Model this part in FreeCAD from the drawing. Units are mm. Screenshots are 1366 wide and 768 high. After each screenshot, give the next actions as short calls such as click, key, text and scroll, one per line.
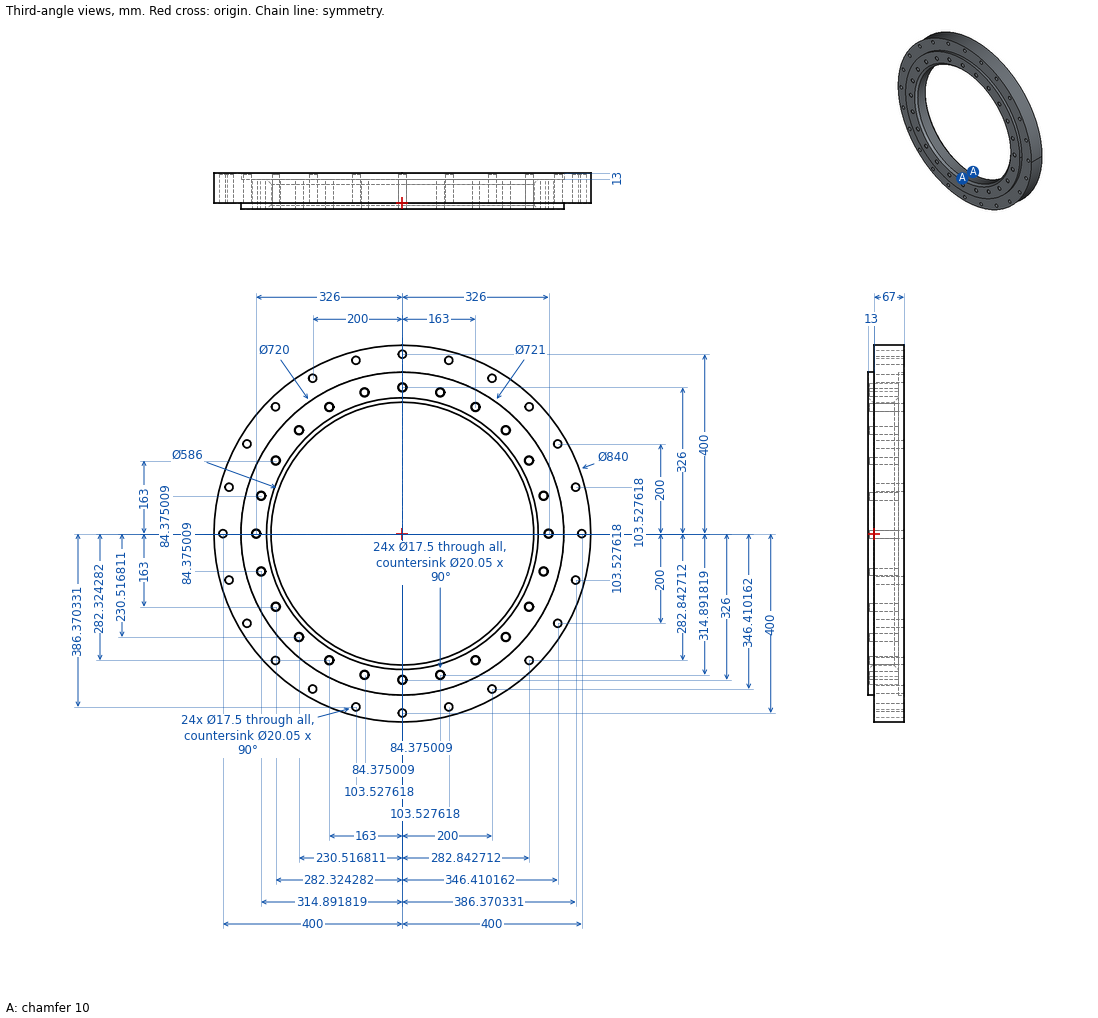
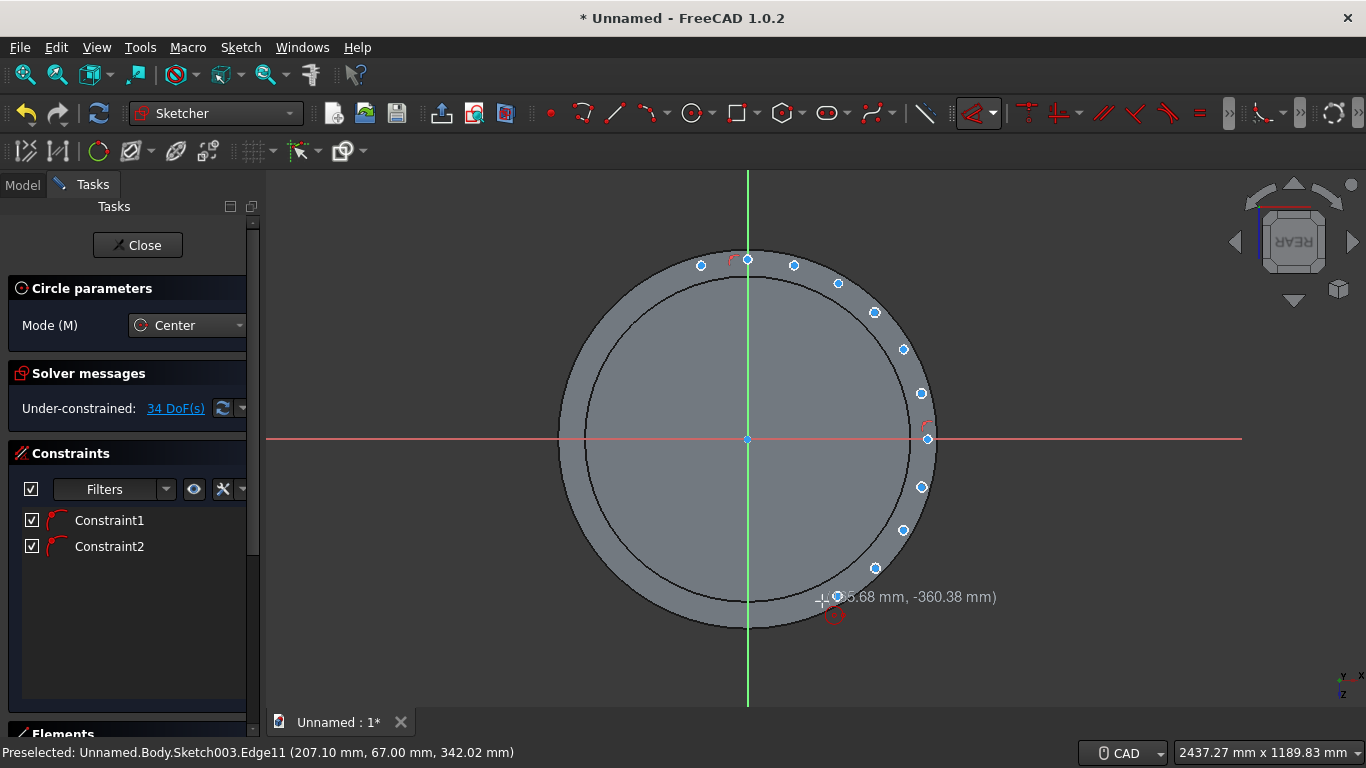
click(794, 614)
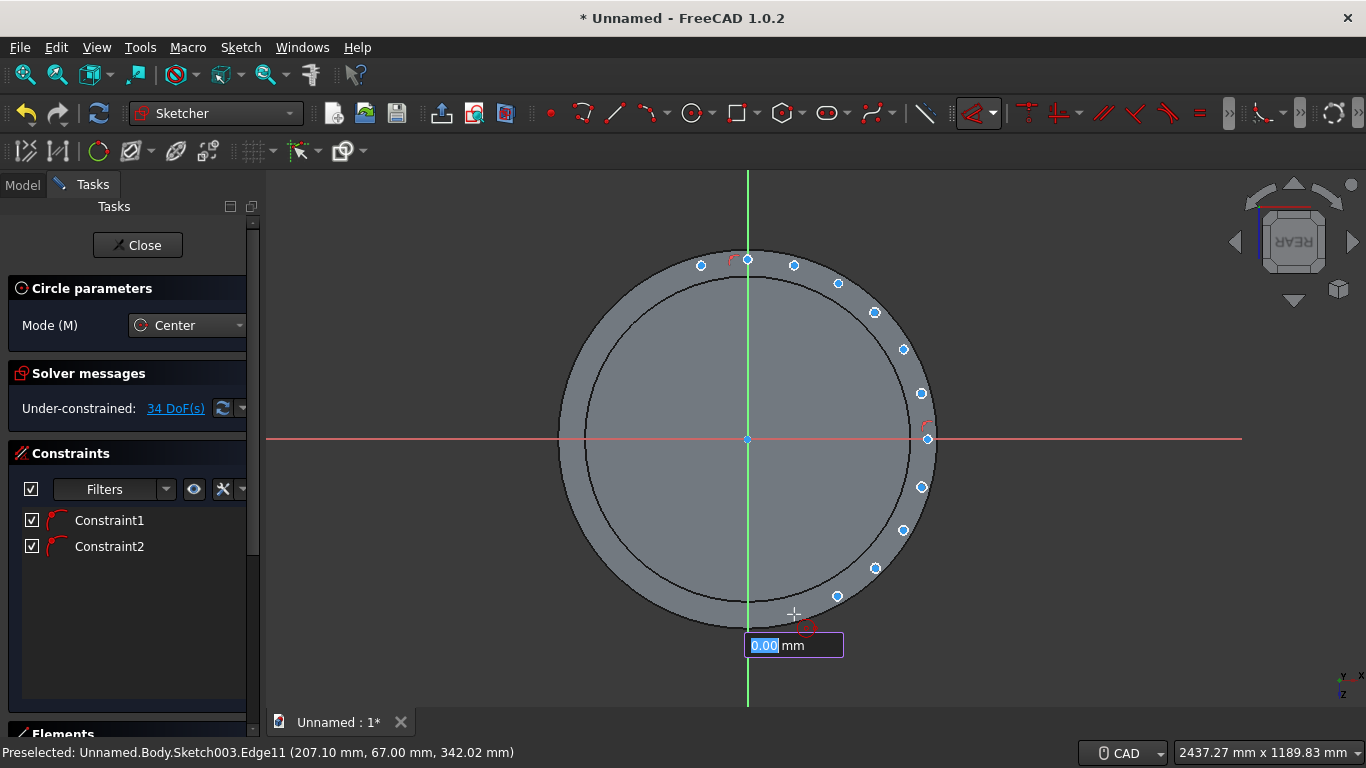
scroll(797, 611, up, 7)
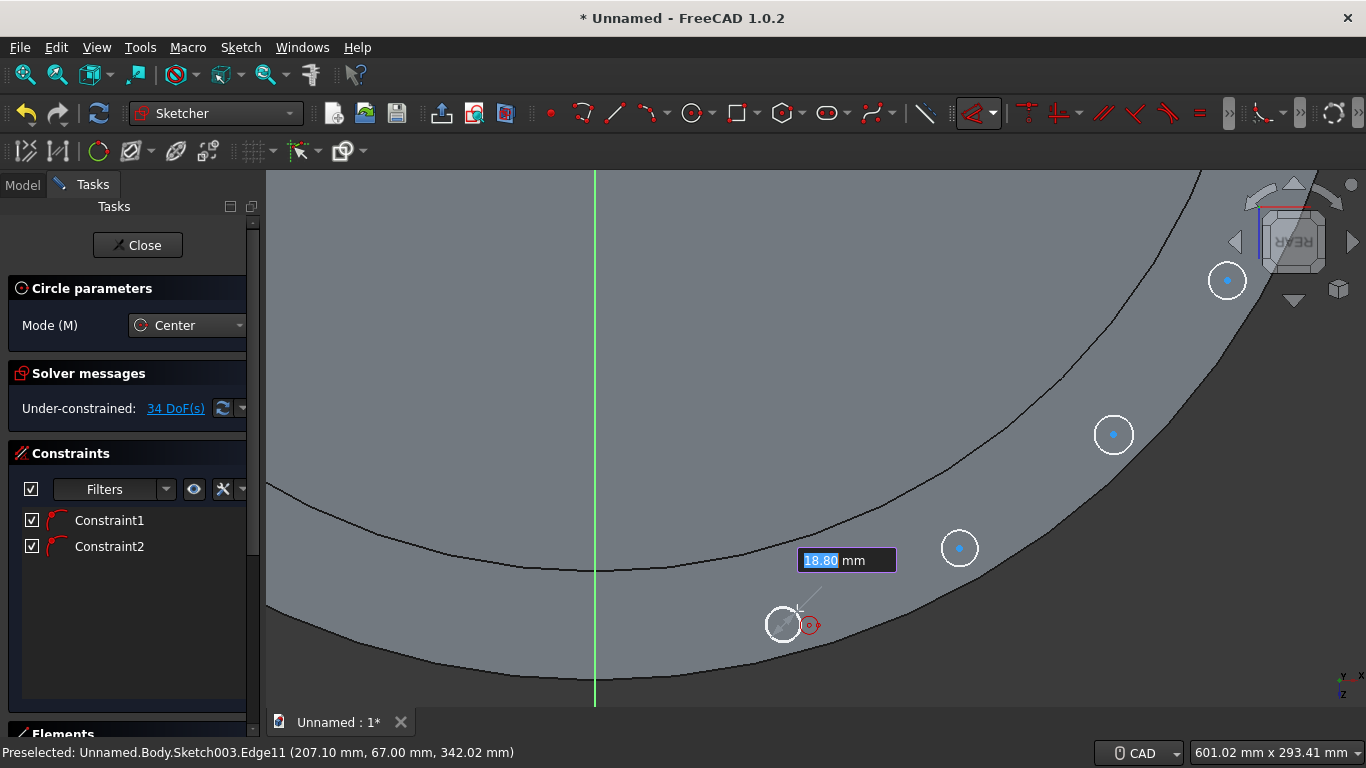
click(796, 608)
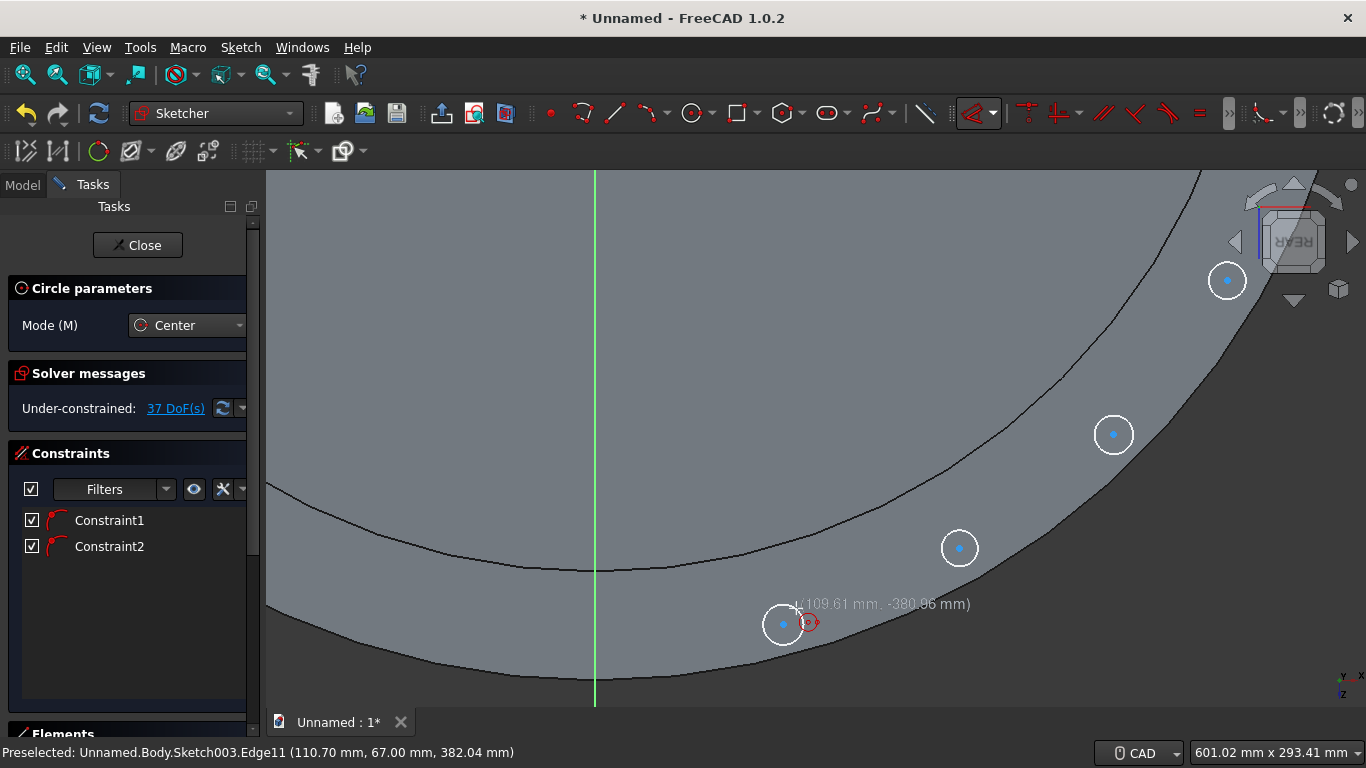
scroll(595, 644, up, 2)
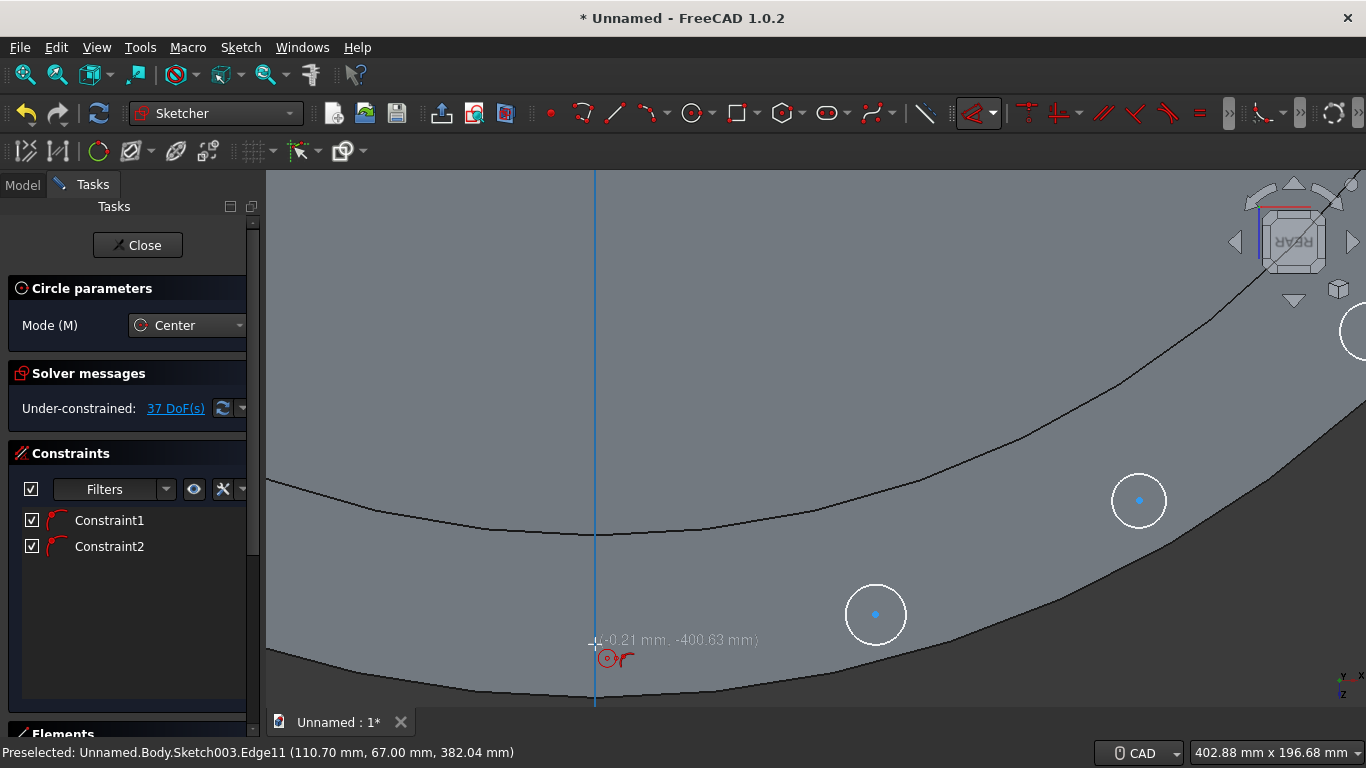
scroll(778, 614, down, 9)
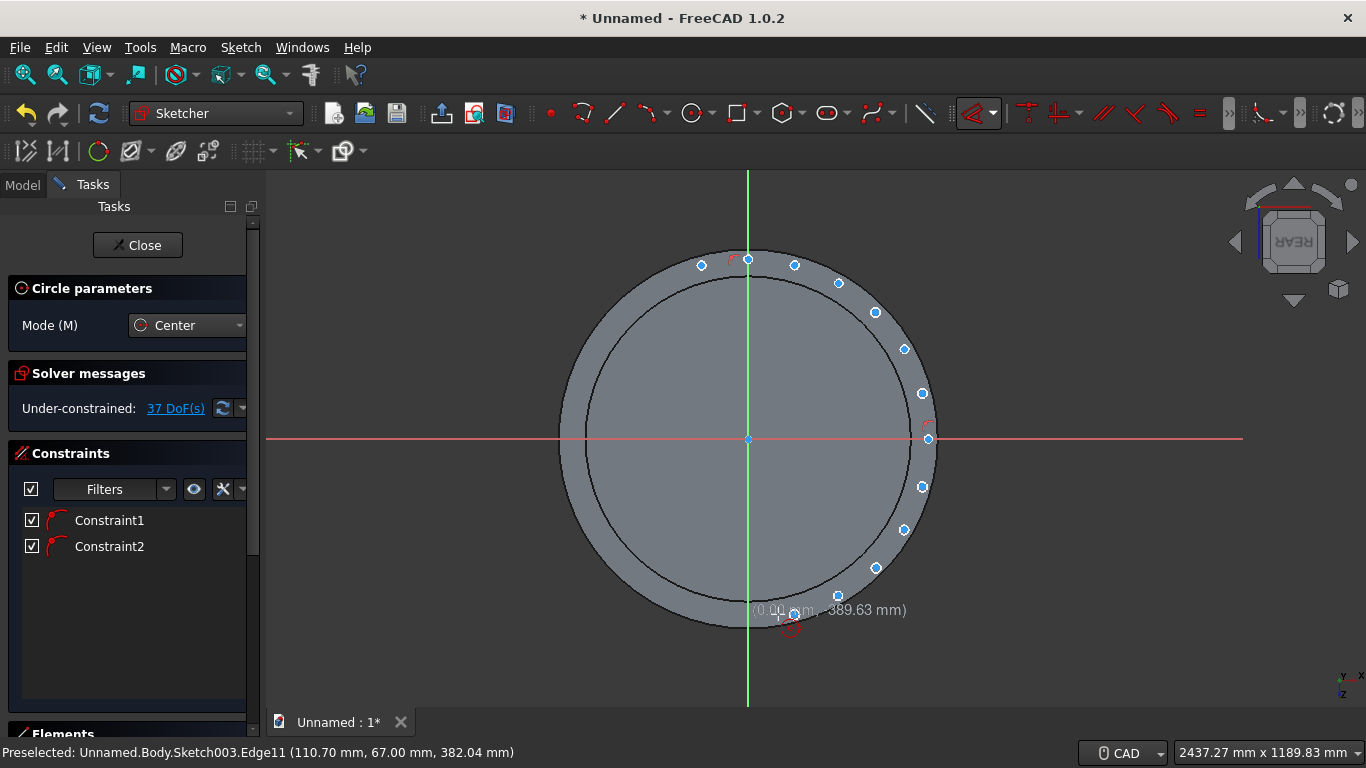
click(748, 620)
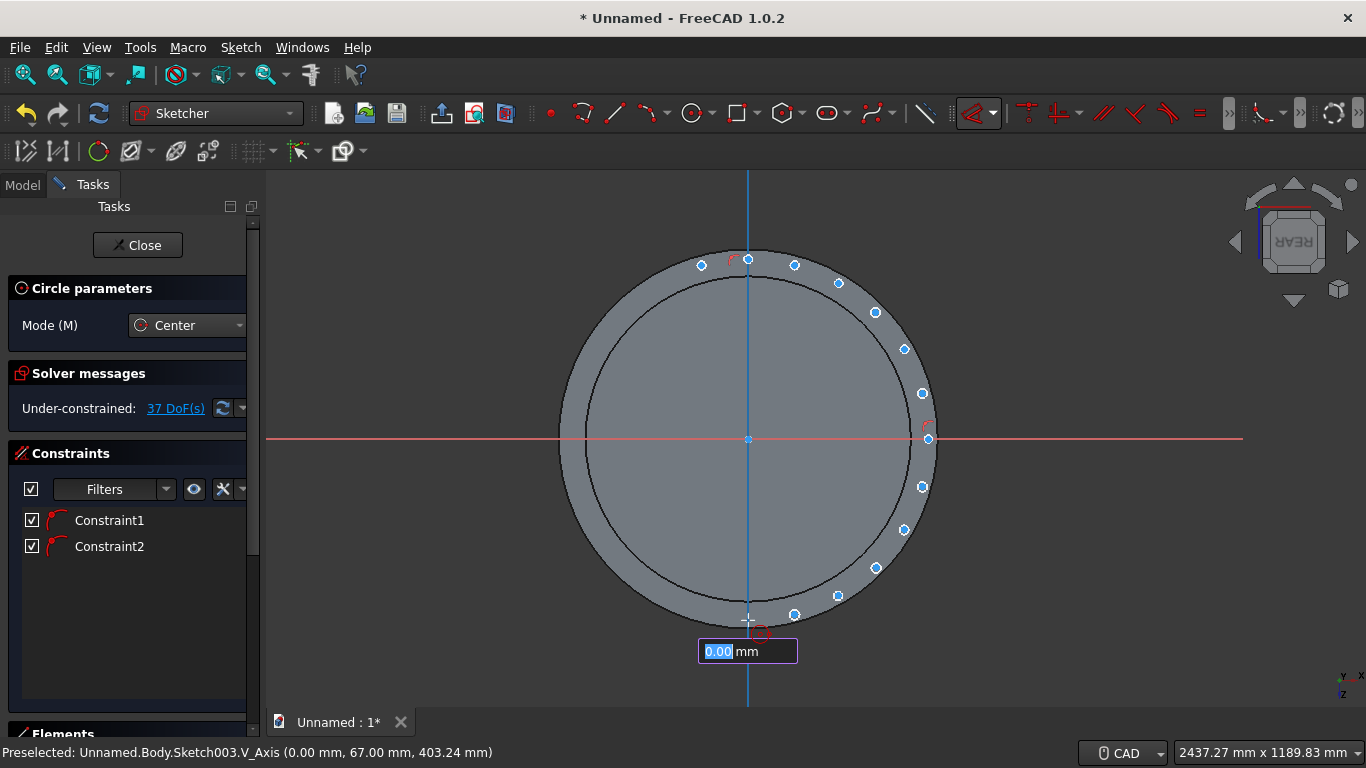
scroll(752, 618, up, 8)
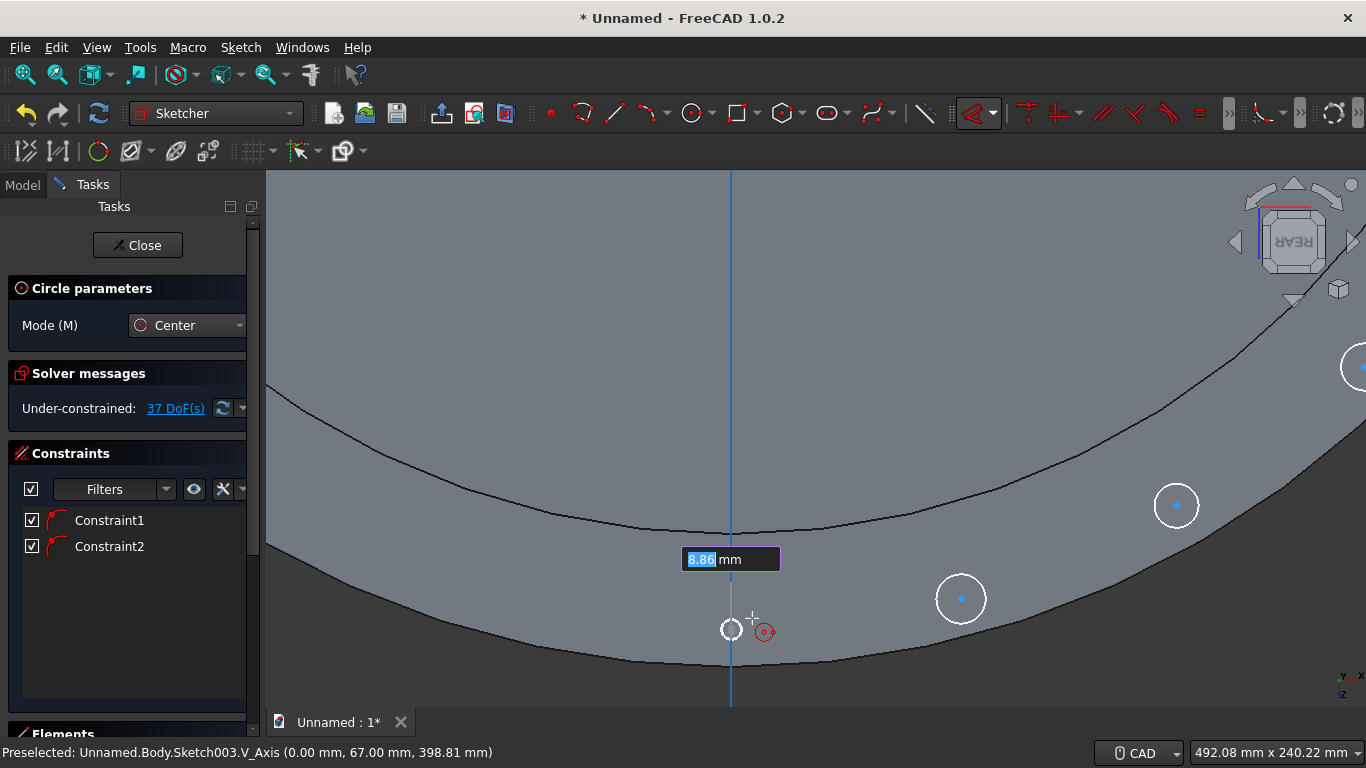
click(750, 616)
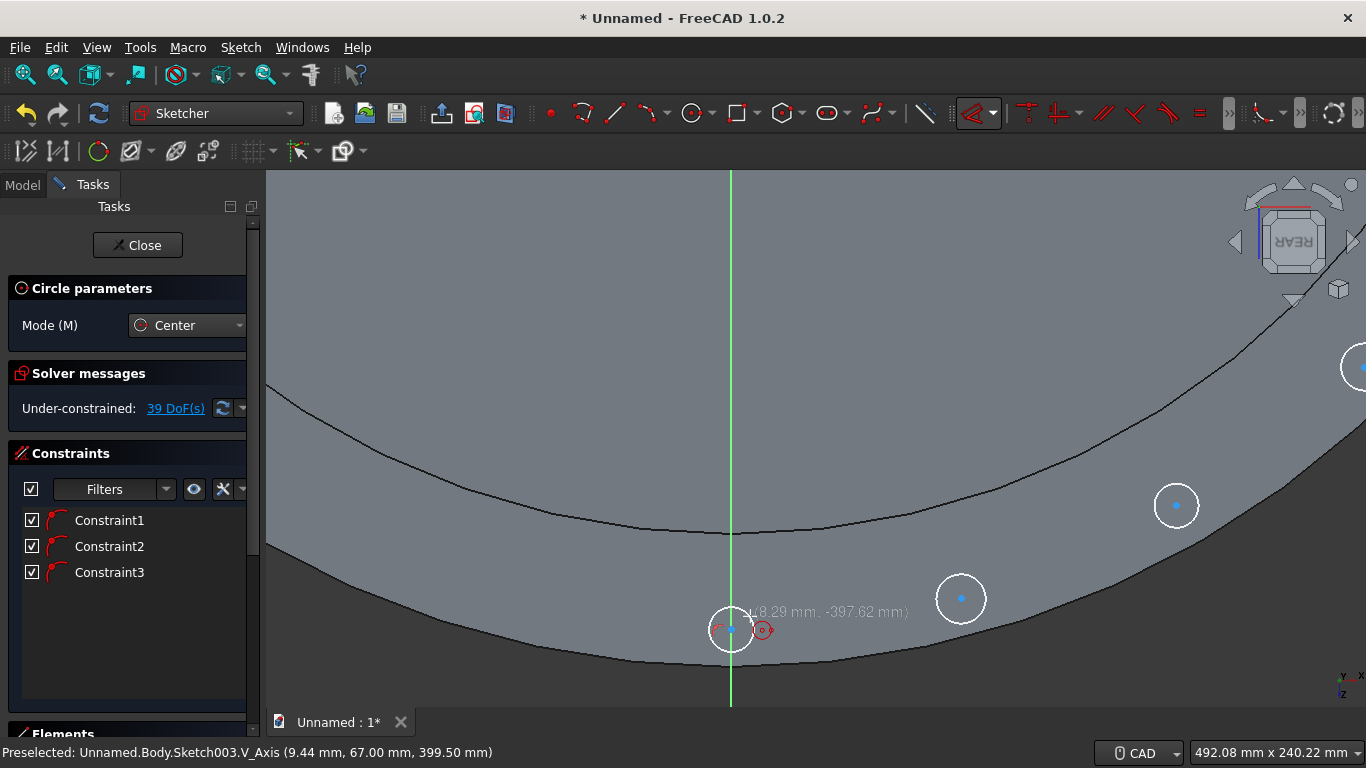
scroll(752, 618, down, 8)